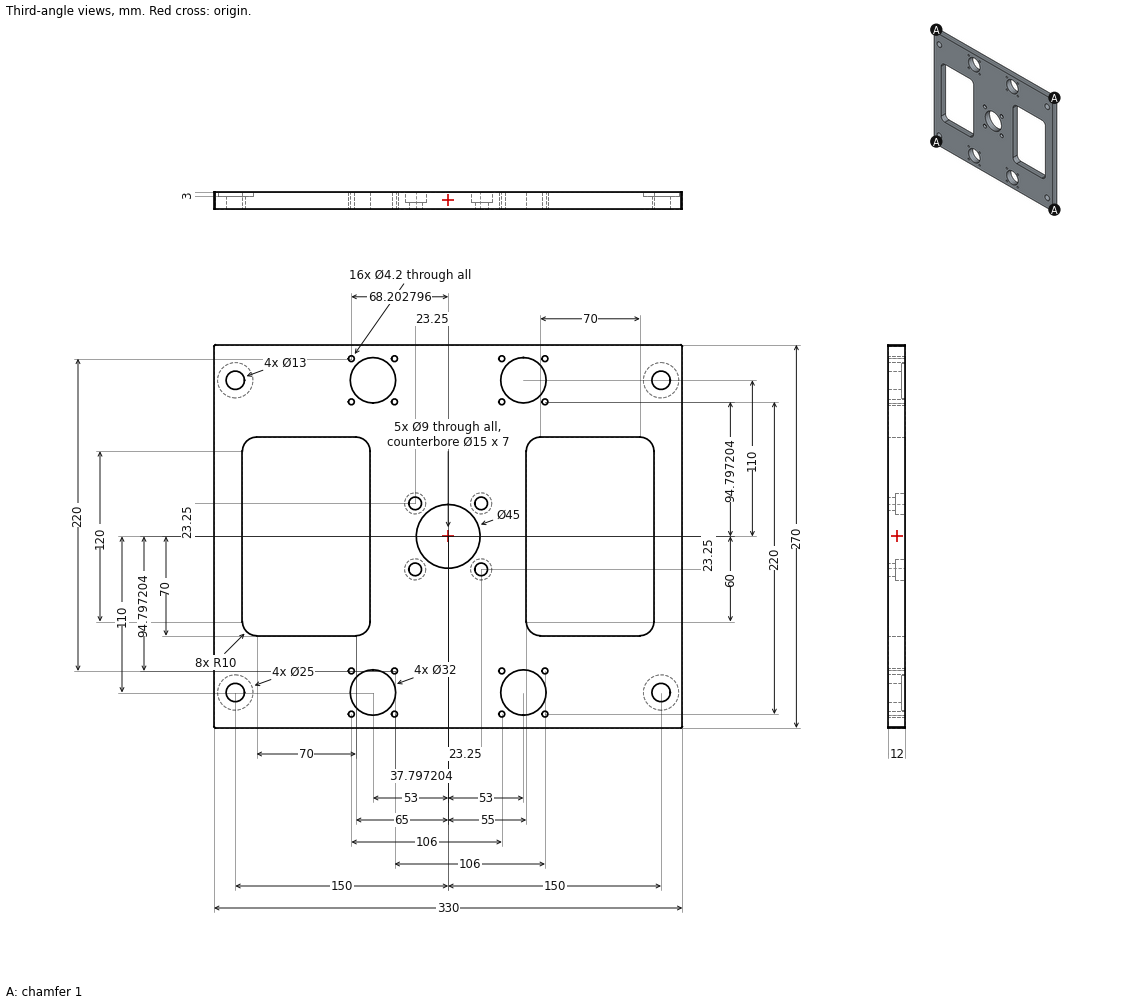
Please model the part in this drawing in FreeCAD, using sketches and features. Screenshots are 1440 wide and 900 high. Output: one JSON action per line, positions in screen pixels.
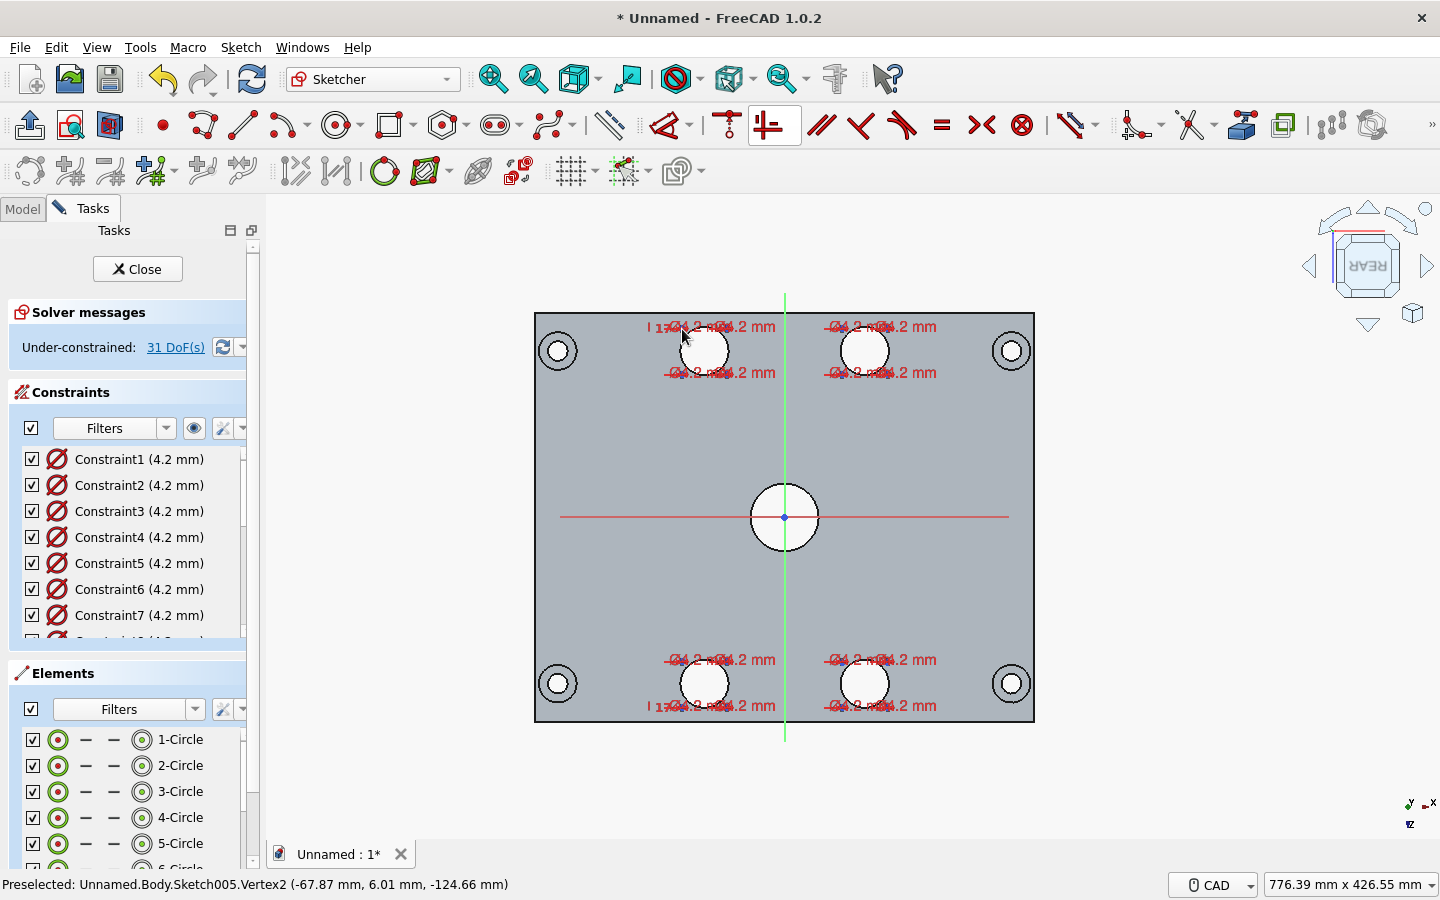
{"action": "left_click", "coordinate": [682, 329]}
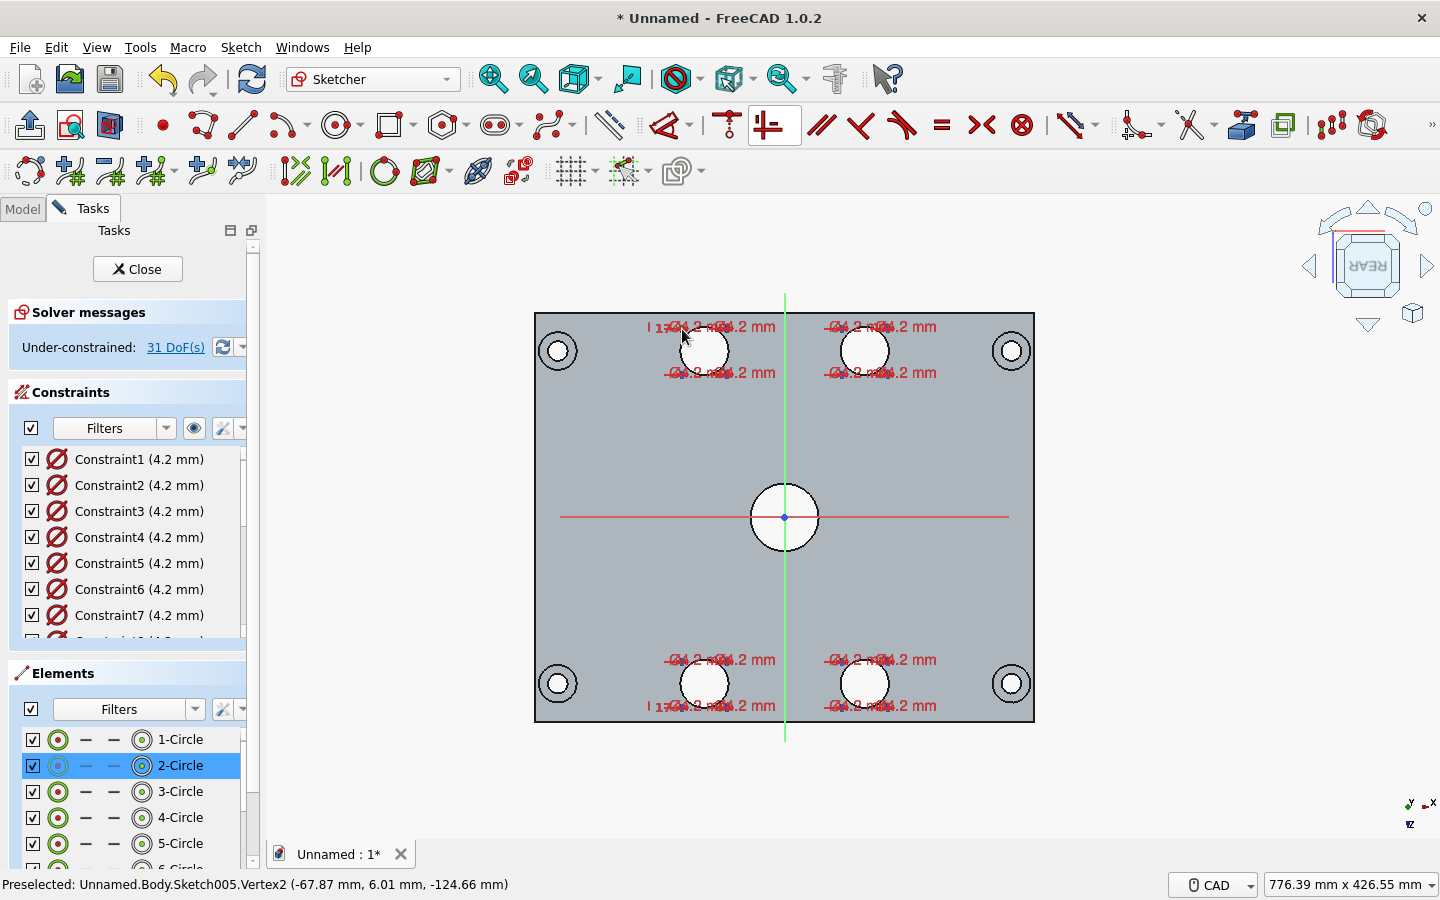
{"action": "left_click", "coordinate": [727, 329]}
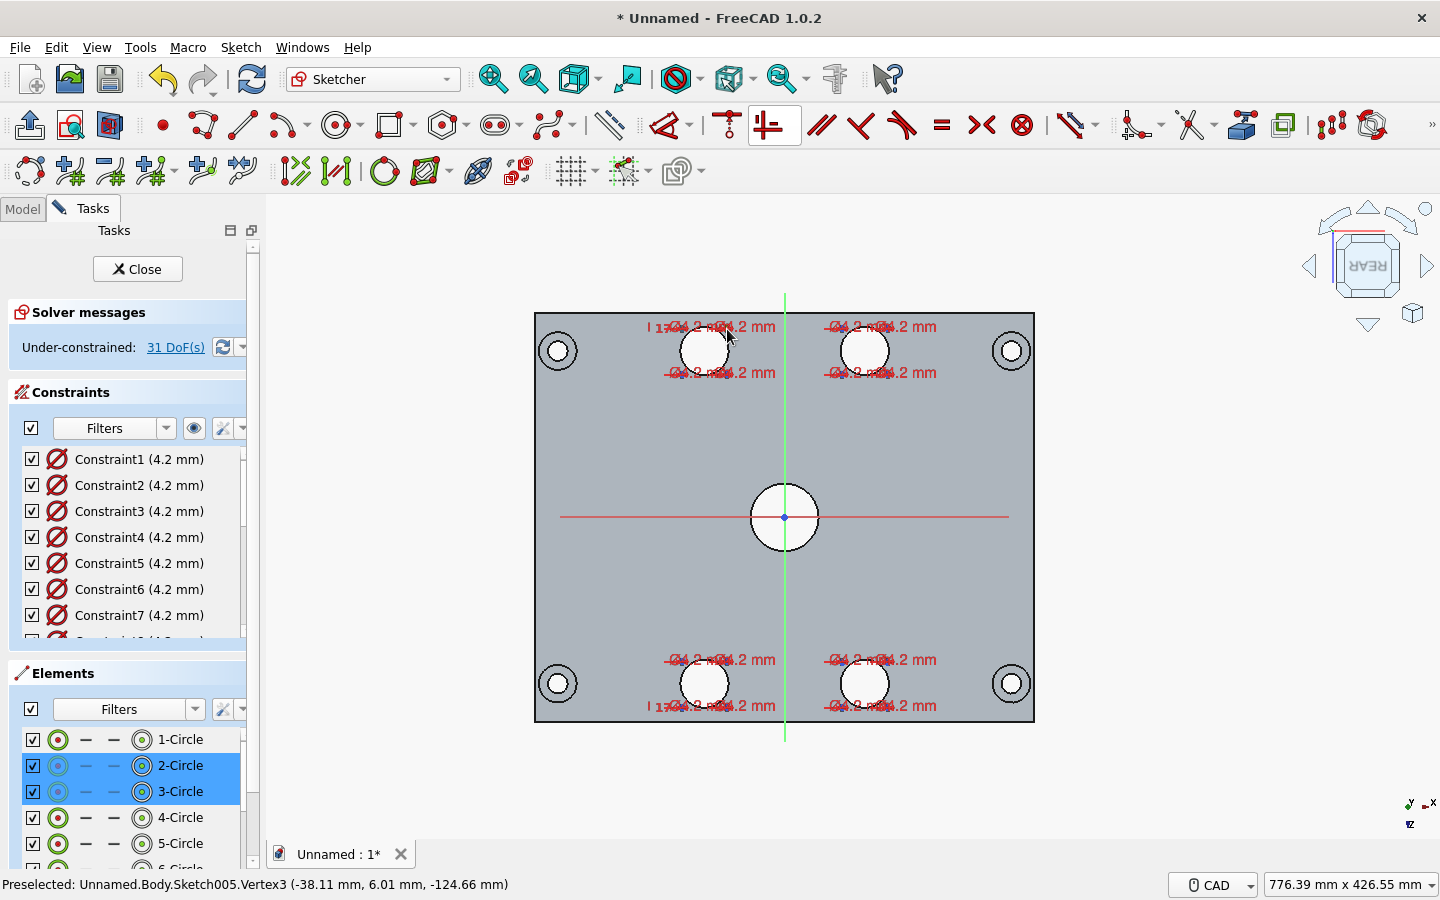
{"action": "key", "text": "h"}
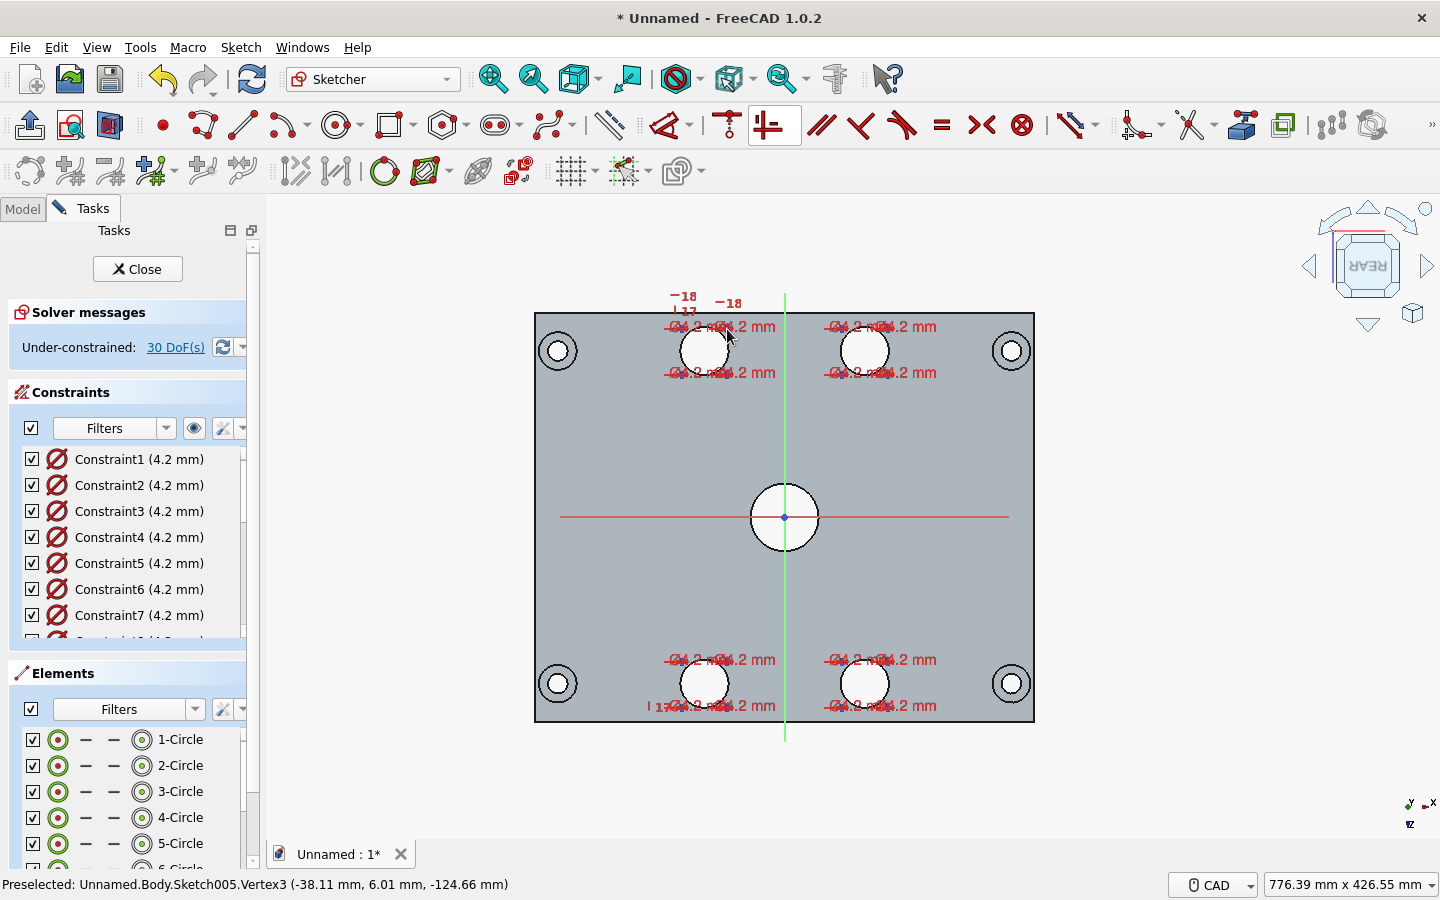
{"action": "left_click", "coordinate": [727, 329]}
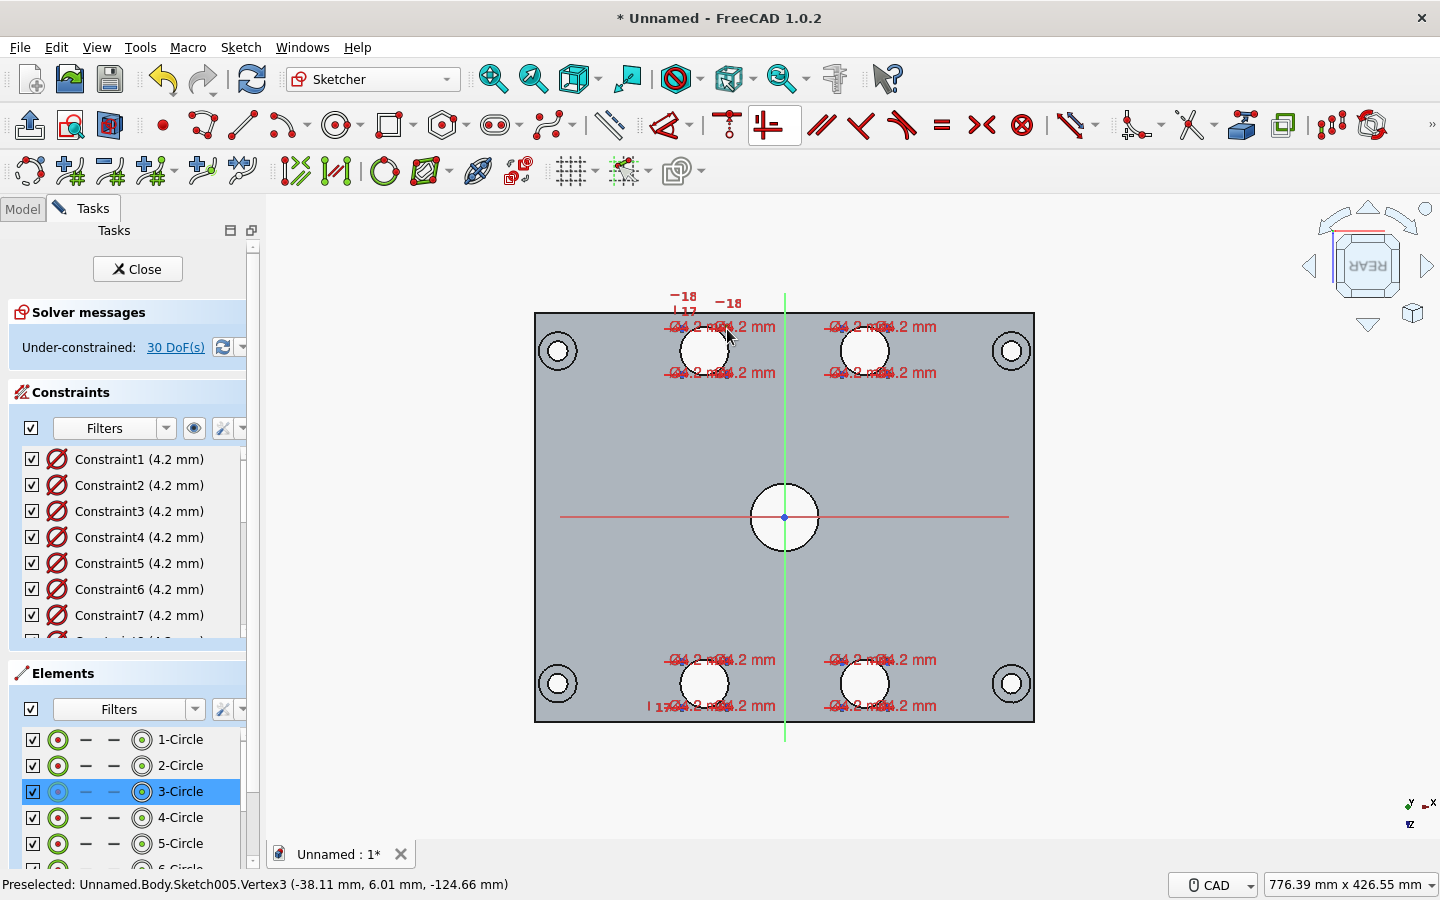
{"action": "left_click", "coordinate": [727, 375]}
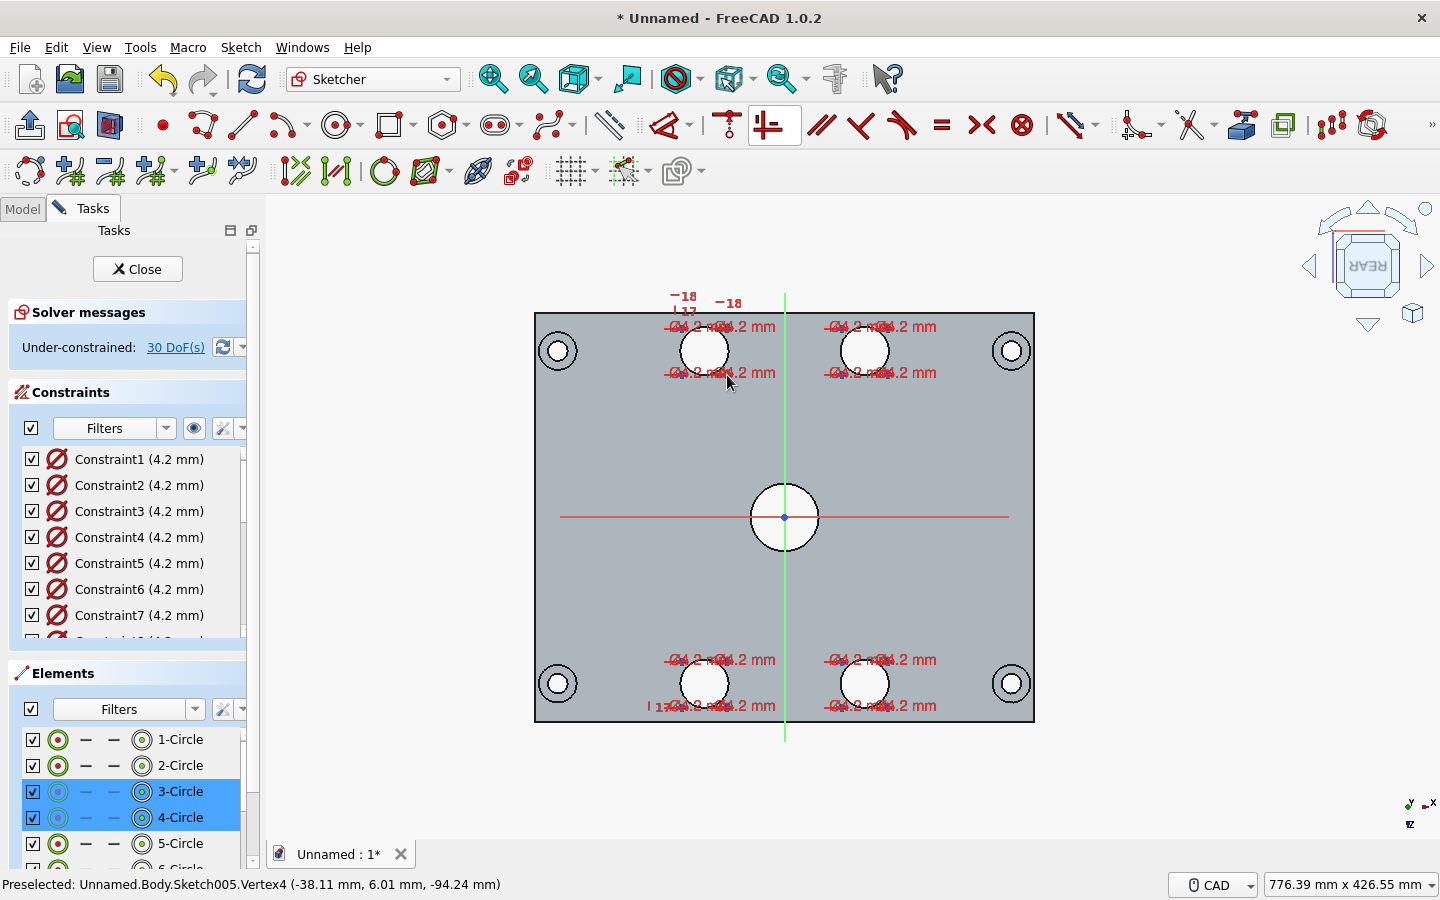
{"action": "left_click", "coordinate": [796, 126]}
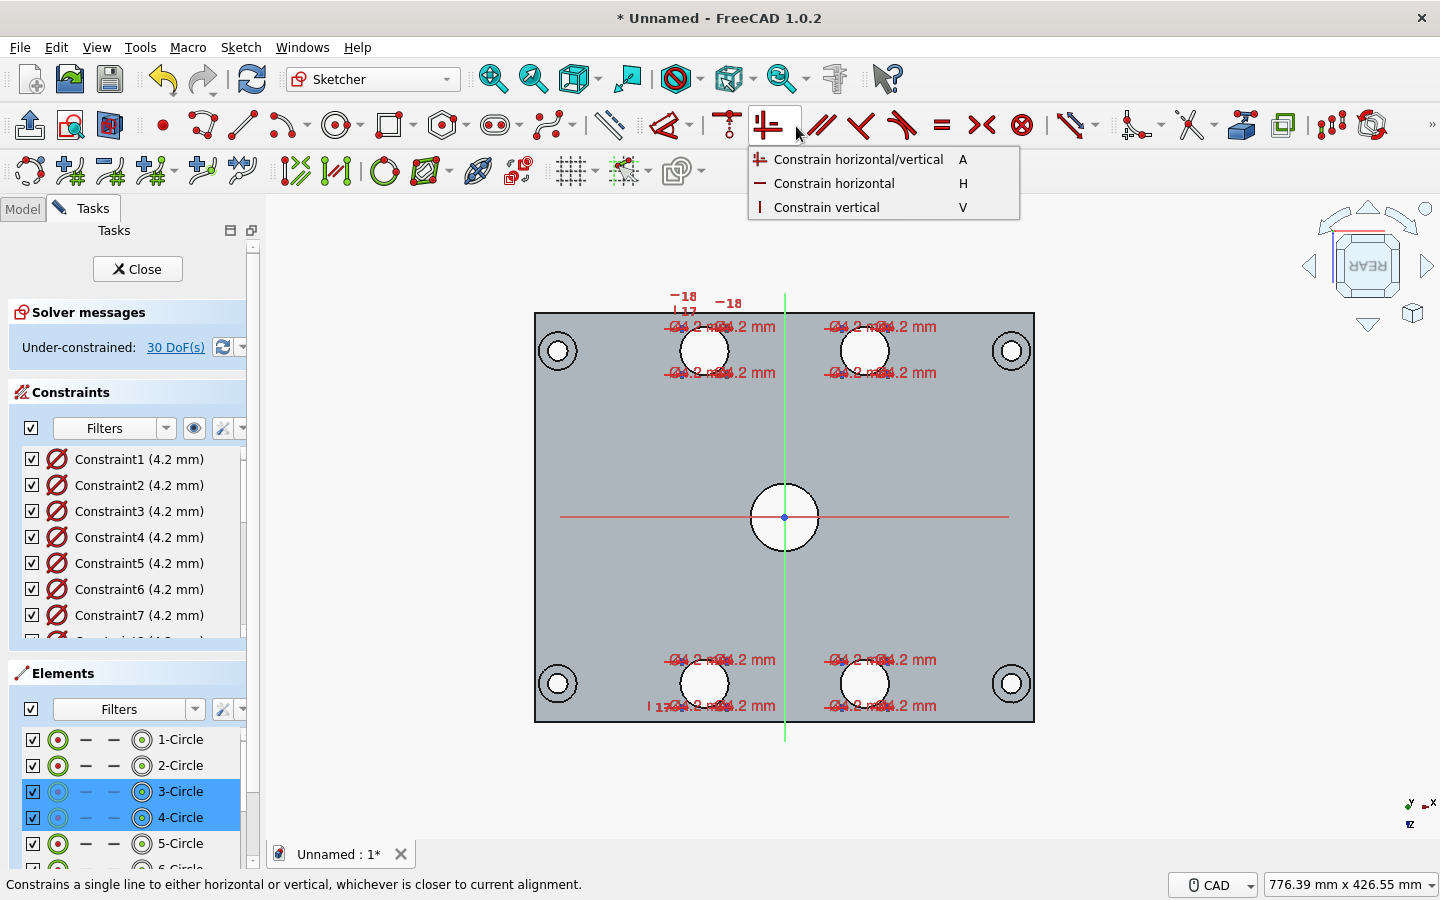
{"action": "left_click", "coordinate": [884, 207]}